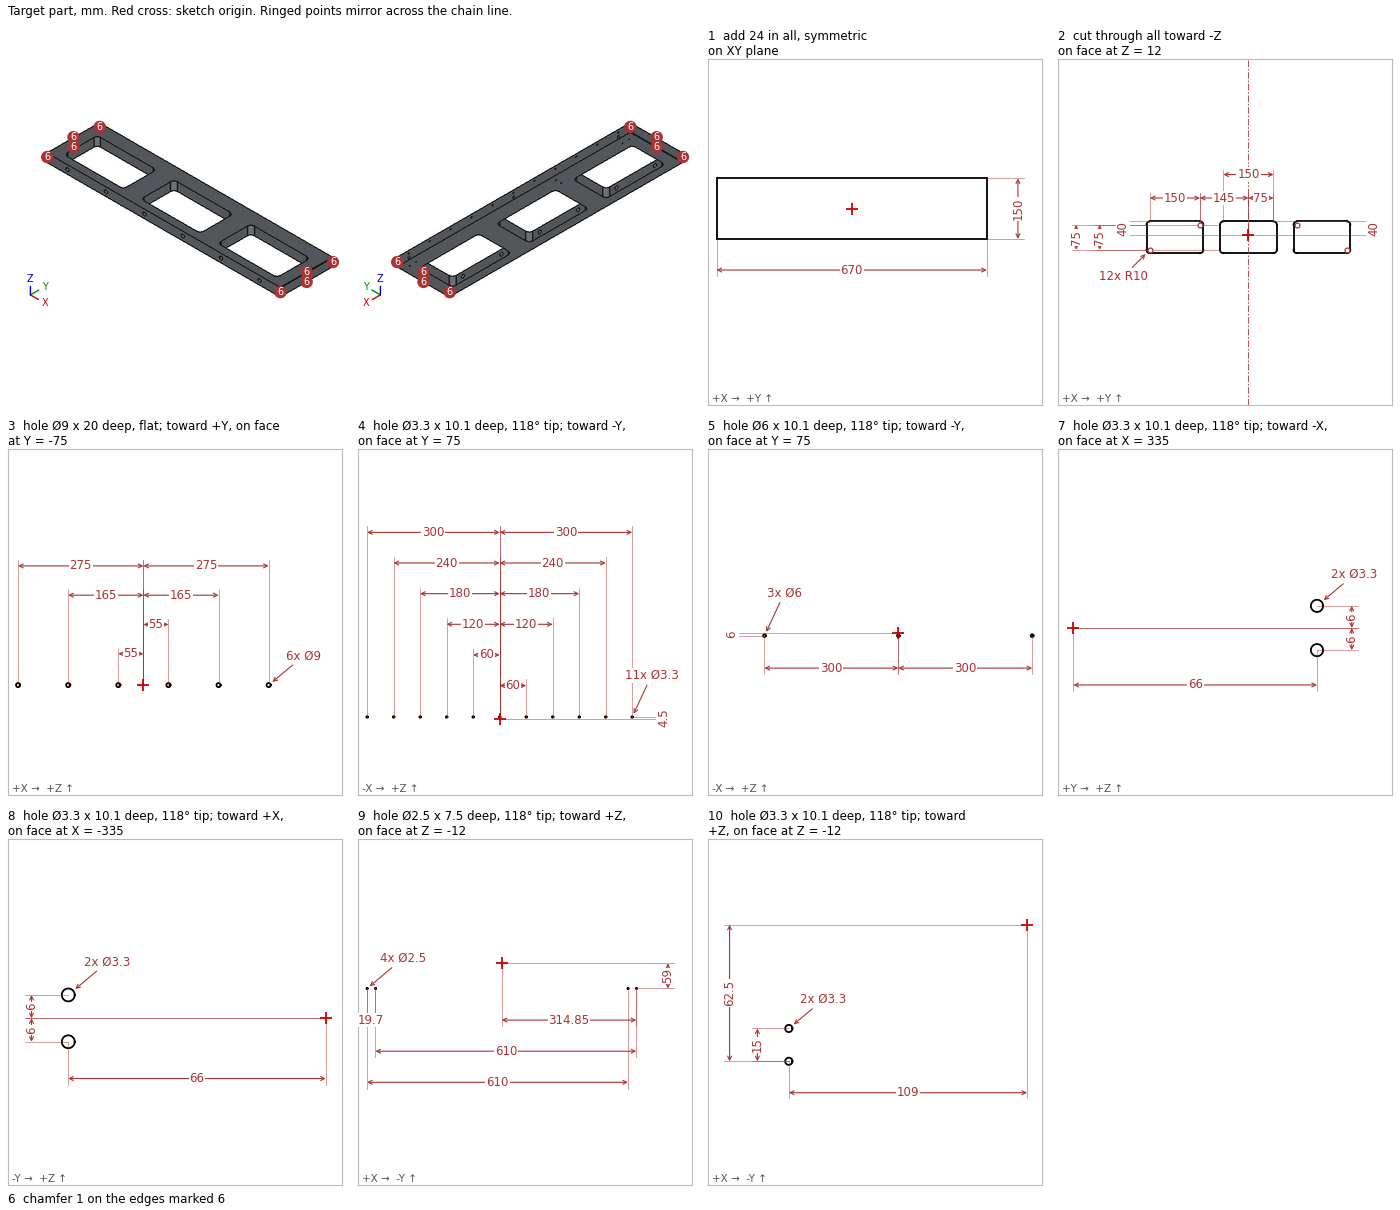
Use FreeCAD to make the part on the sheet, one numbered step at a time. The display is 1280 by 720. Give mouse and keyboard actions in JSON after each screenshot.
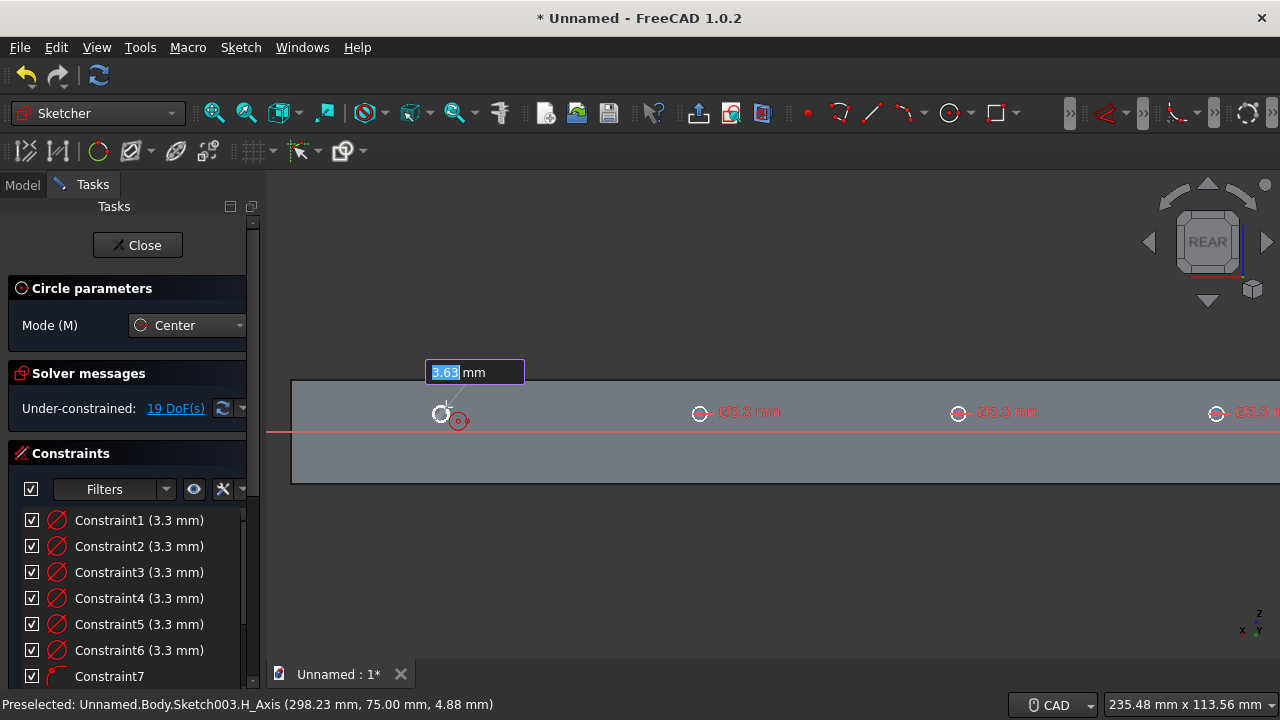
{"action": "type", "text": "3.3"}
{"action": "key", "text": "Return"}
{"action": "key", "text": "Escape"}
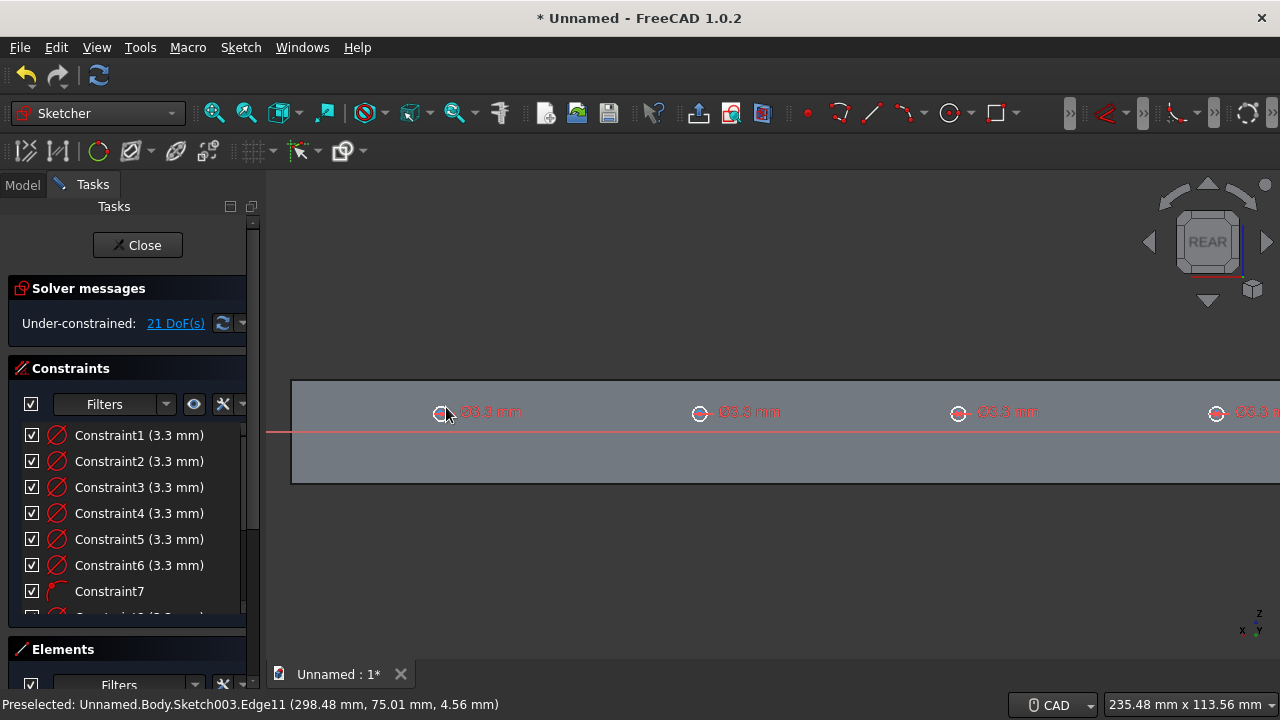
{"action": "scroll", "coordinate": [444, 413], "scroll_direction": "down", "scroll_amount": 8}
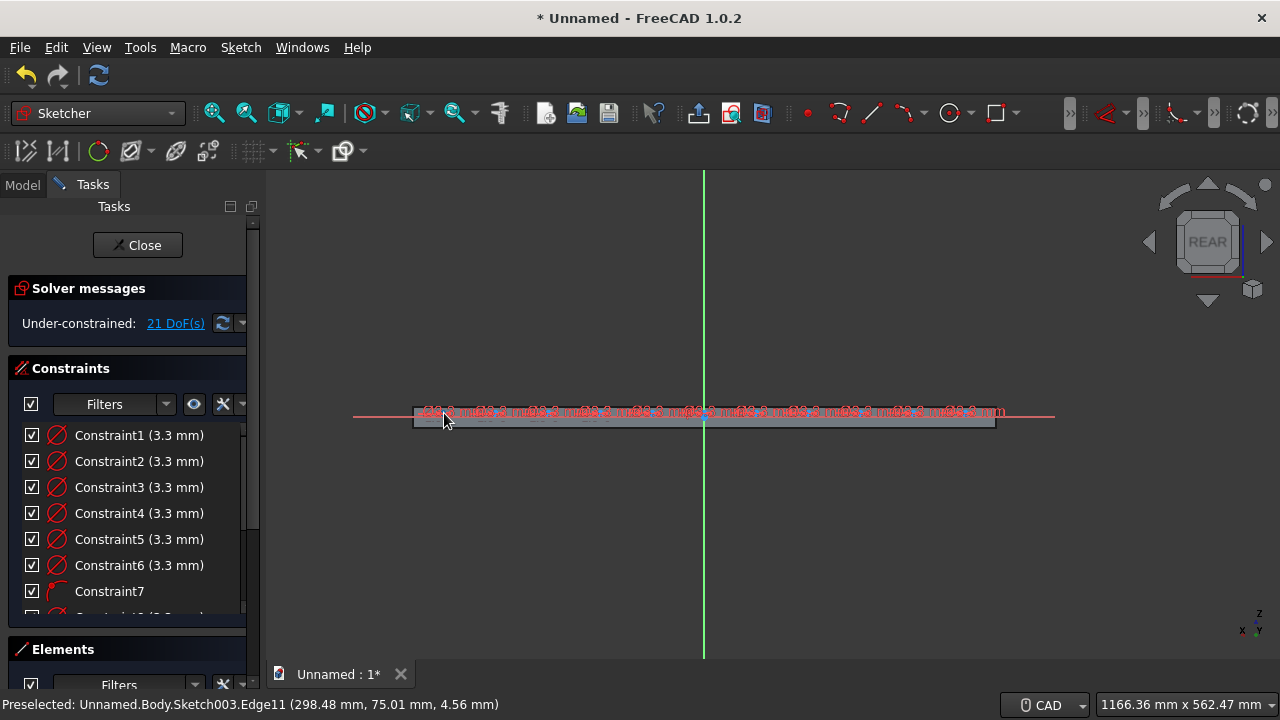
{"action": "left_click", "coordinate": [965, 413]}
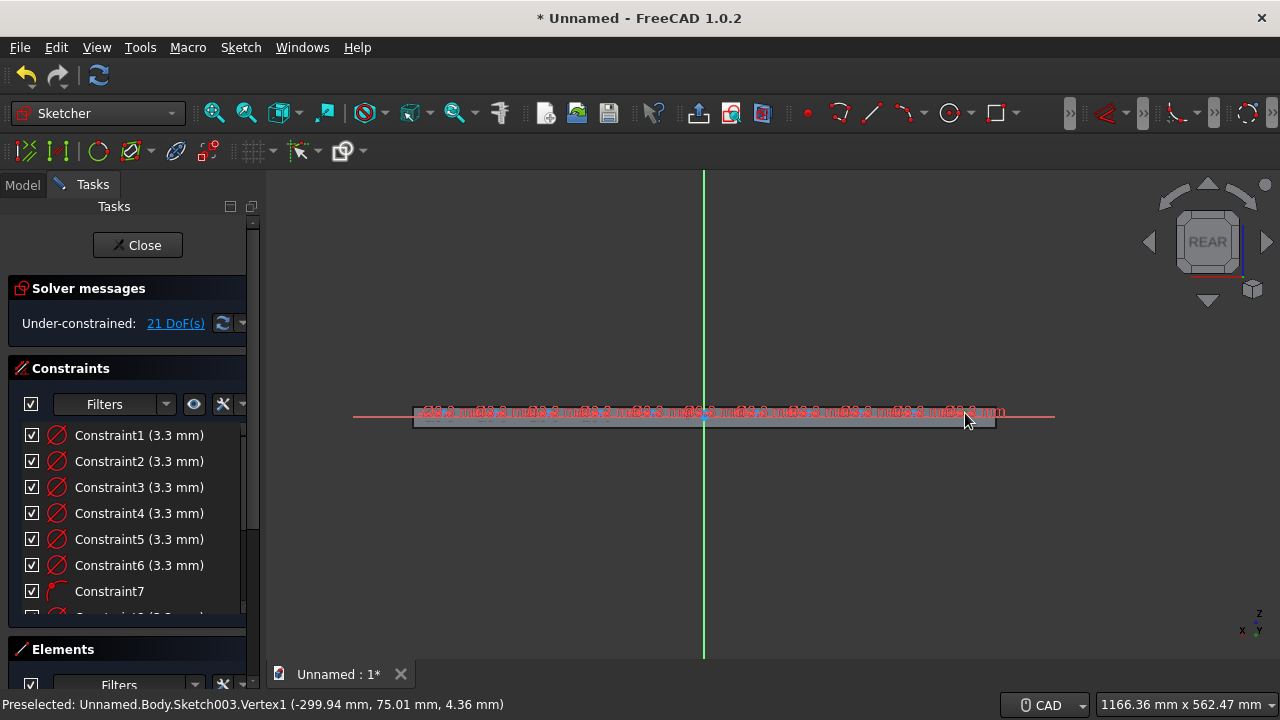
{"action": "left_click", "coordinate": [913, 413]}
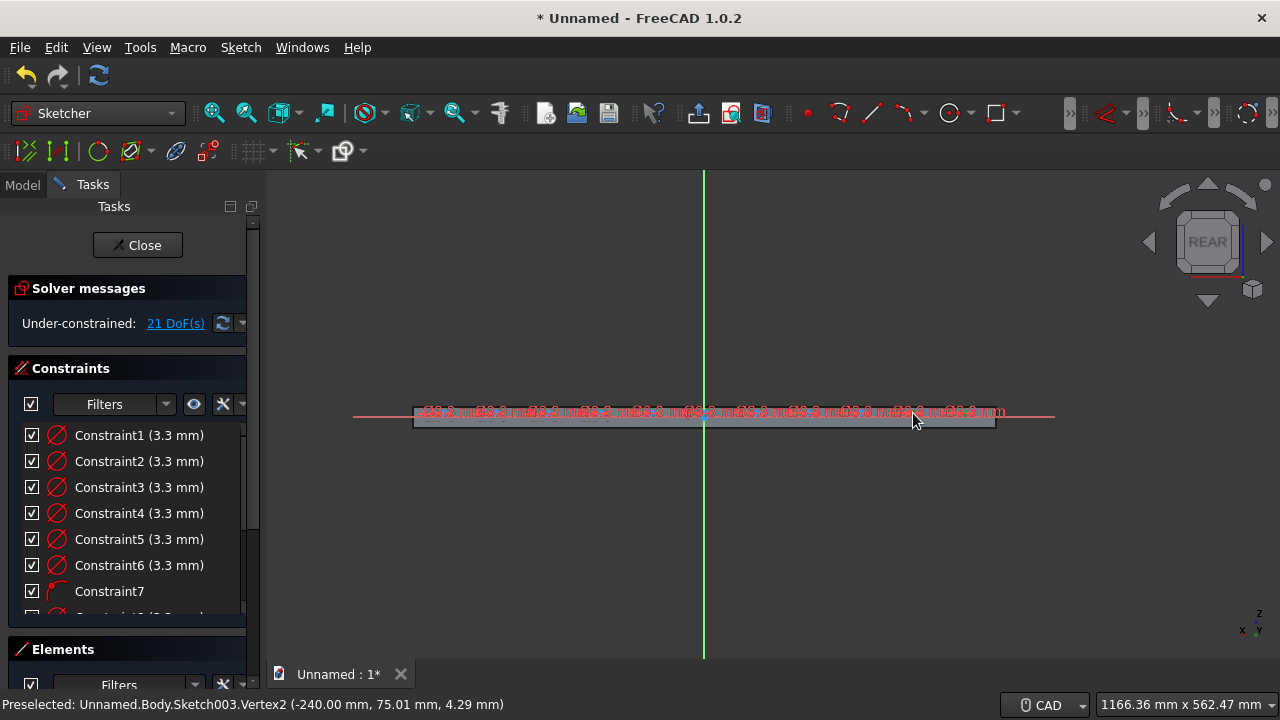
{"action": "key", "text": "h"}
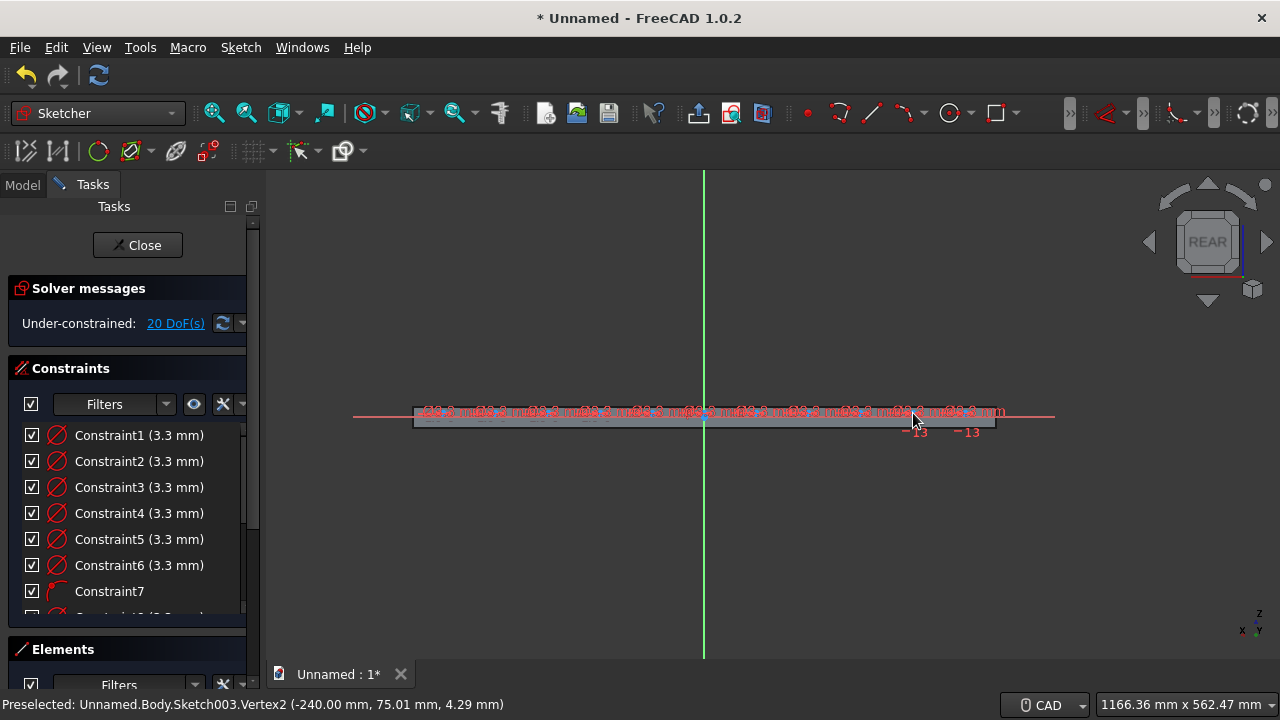
{"action": "left_click", "coordinate": [913, 413]}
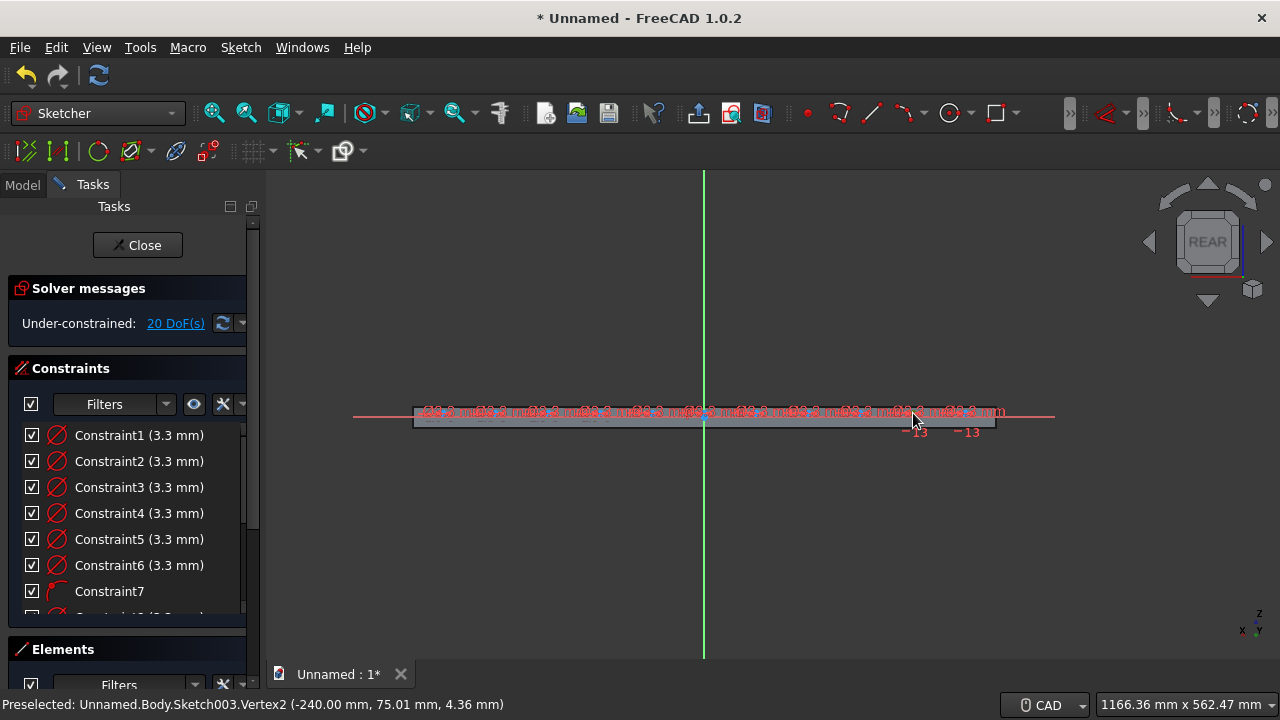
{"action": "left_click", "coordinate": [861, 413]}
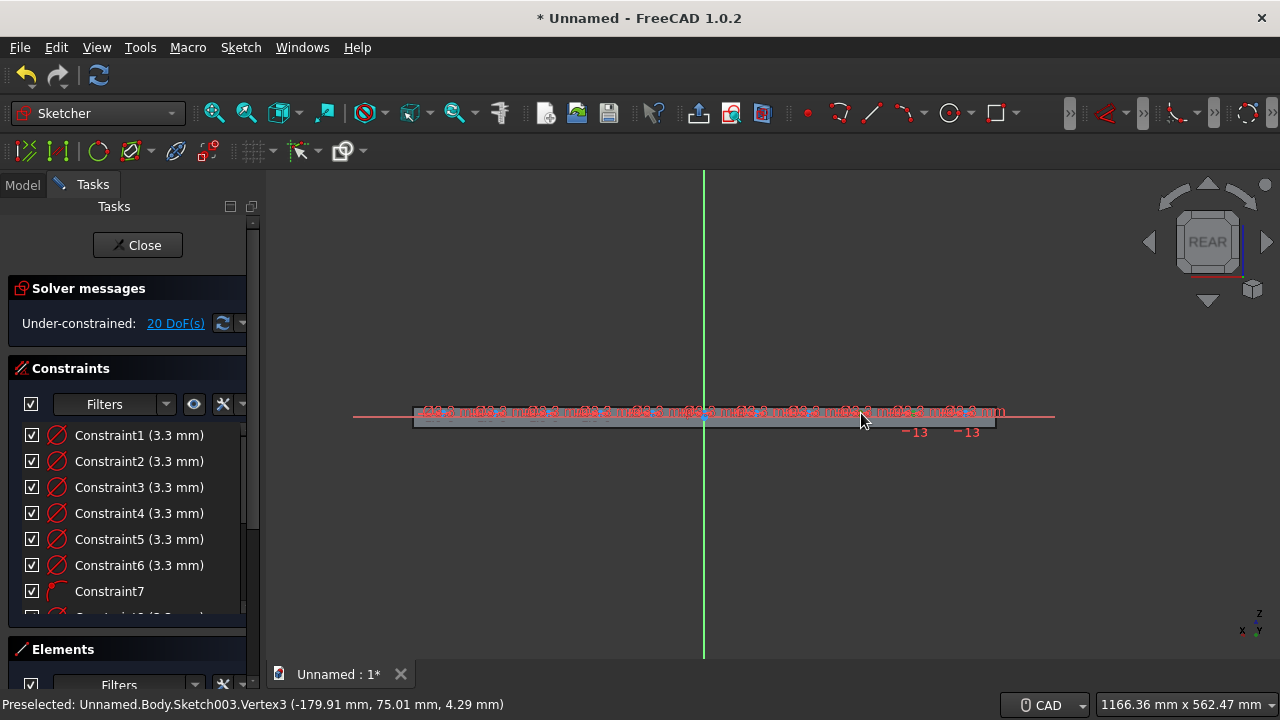
{"action": "key", "text": "h"}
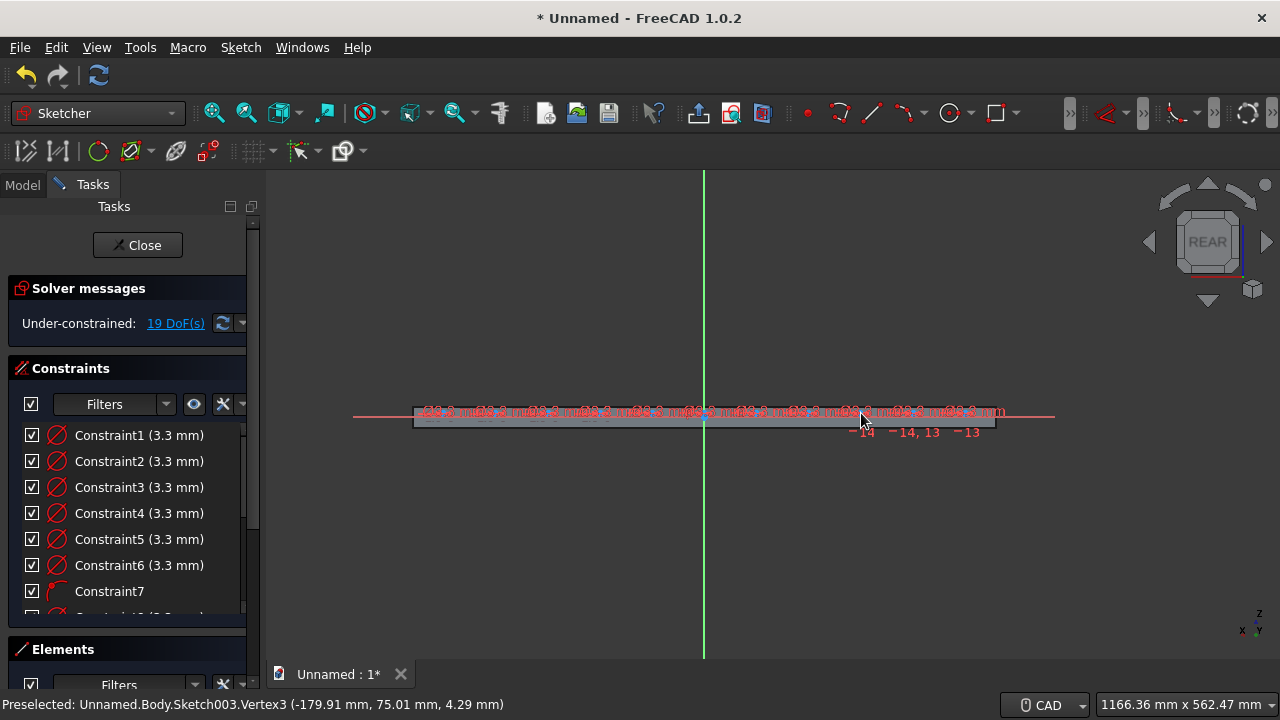
{"action": "left_click", "coordinate": [861, 413]}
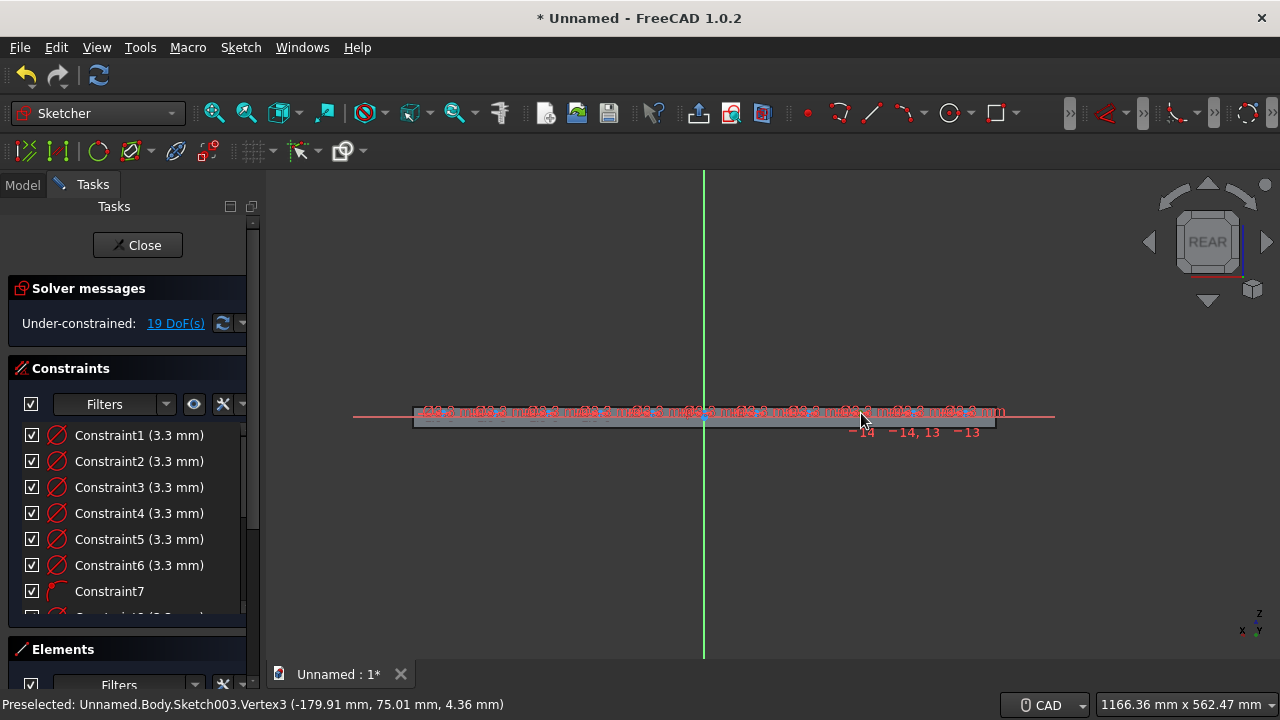
{"action": "left_click", "coordinate": [809, 413]}